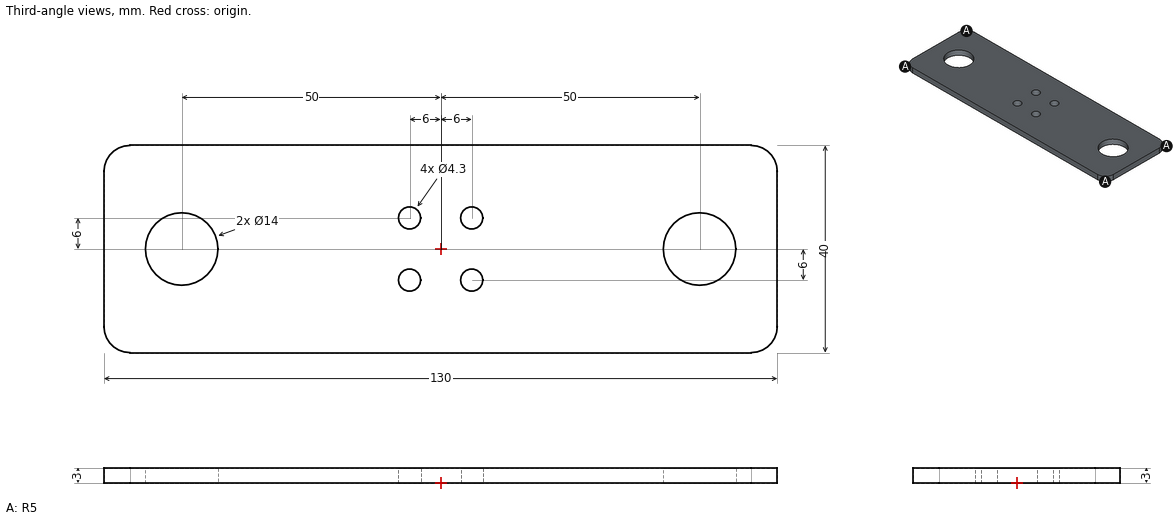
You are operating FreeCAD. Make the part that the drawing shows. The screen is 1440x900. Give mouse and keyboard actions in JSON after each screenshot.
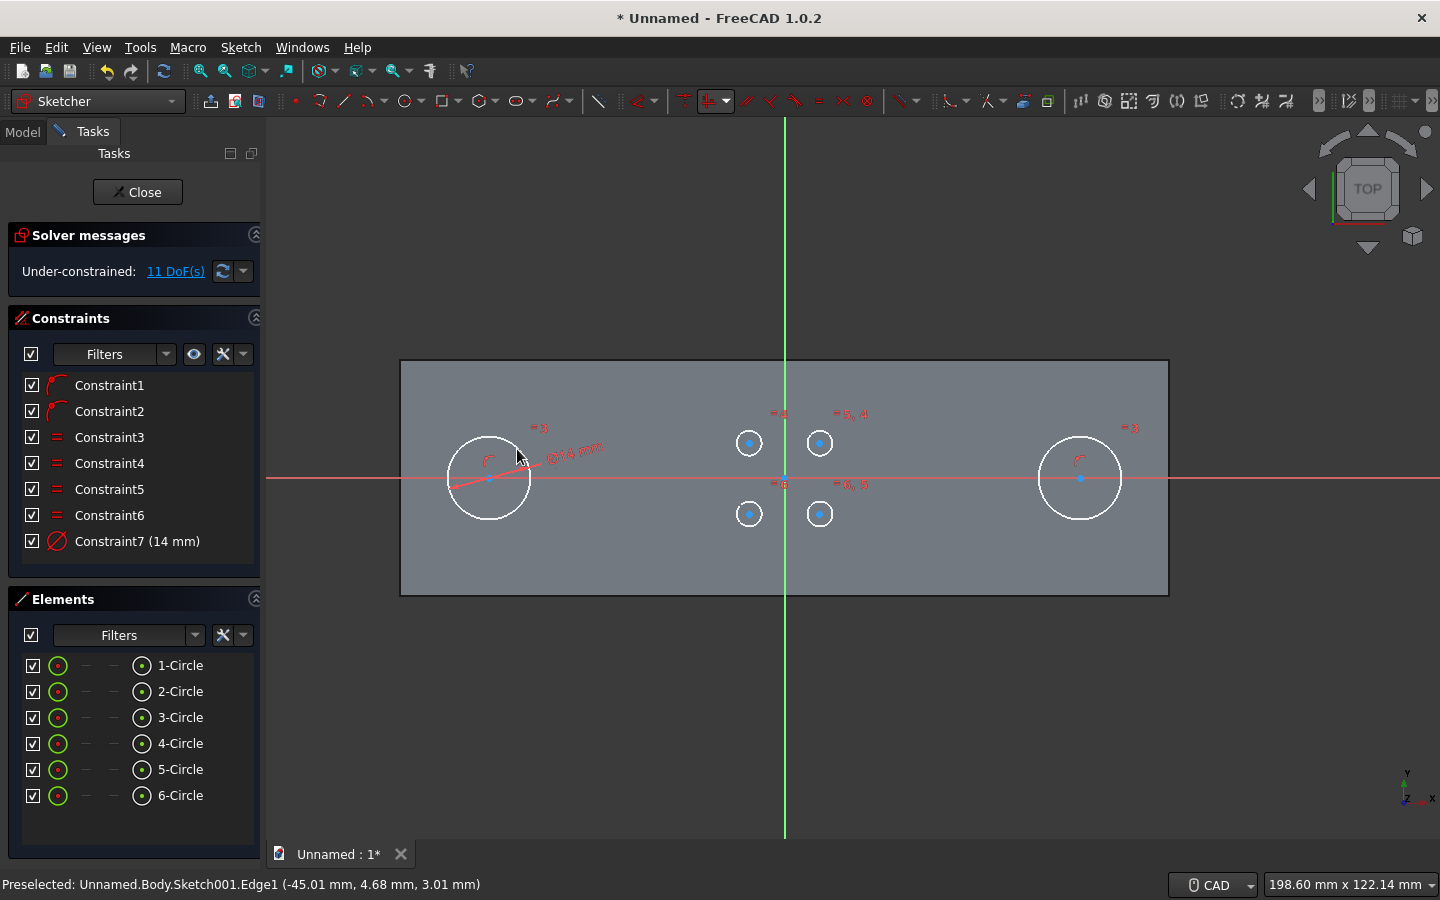
{"action": "scroll", "coordinate": [758, 434], "scroll_direction": "up", "scroll_amount": 3}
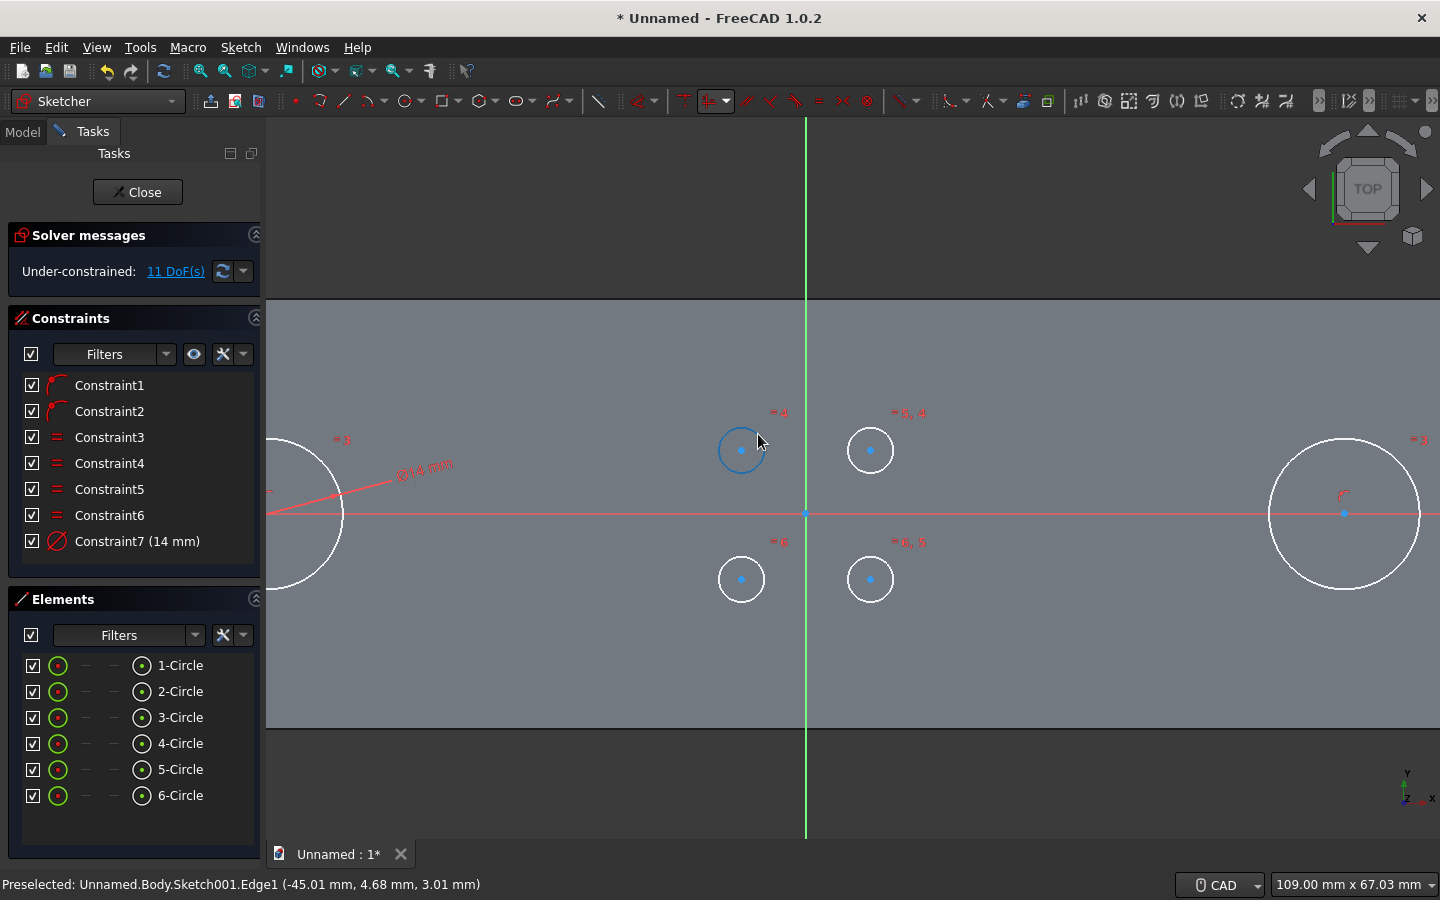
{"action": "left_click", "coordinate": [758, 434]}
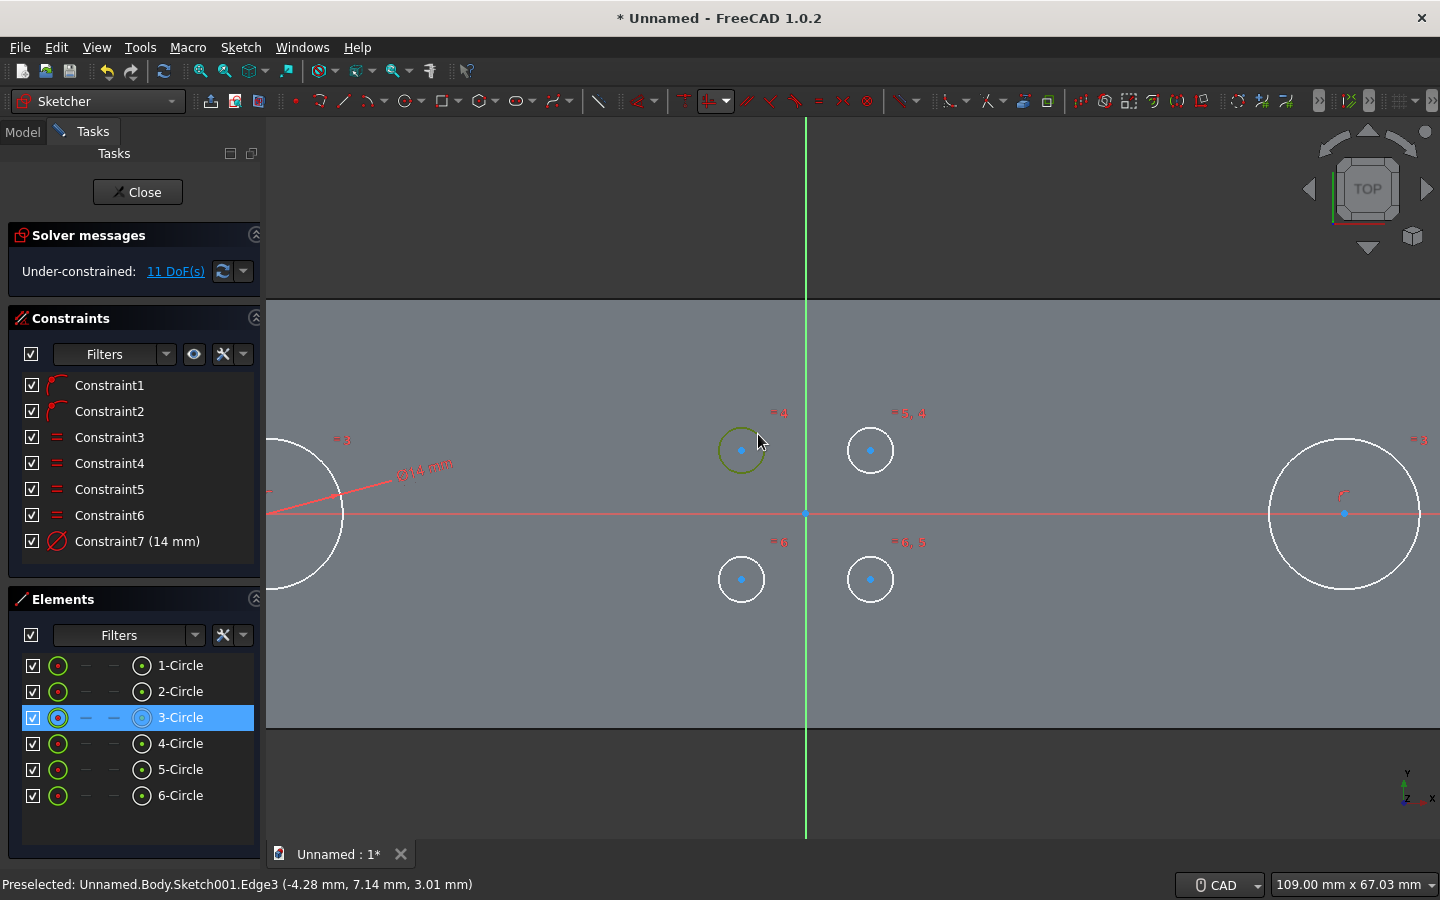
{"action": "key", "text": "k o"}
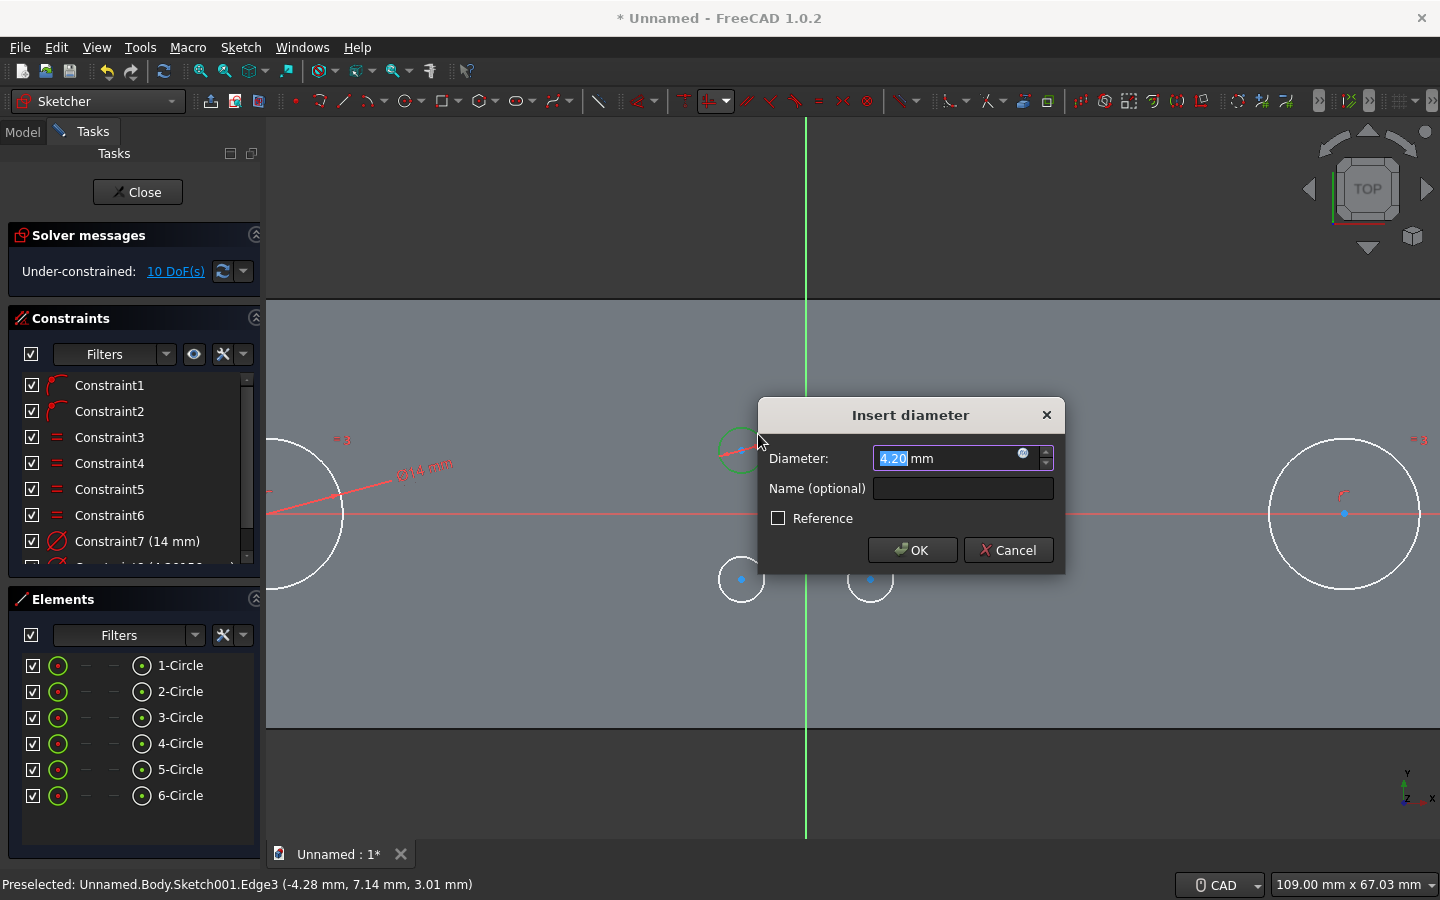
{"action": "type", "text": "4.3"}
{"action": "key", "text": "Return"}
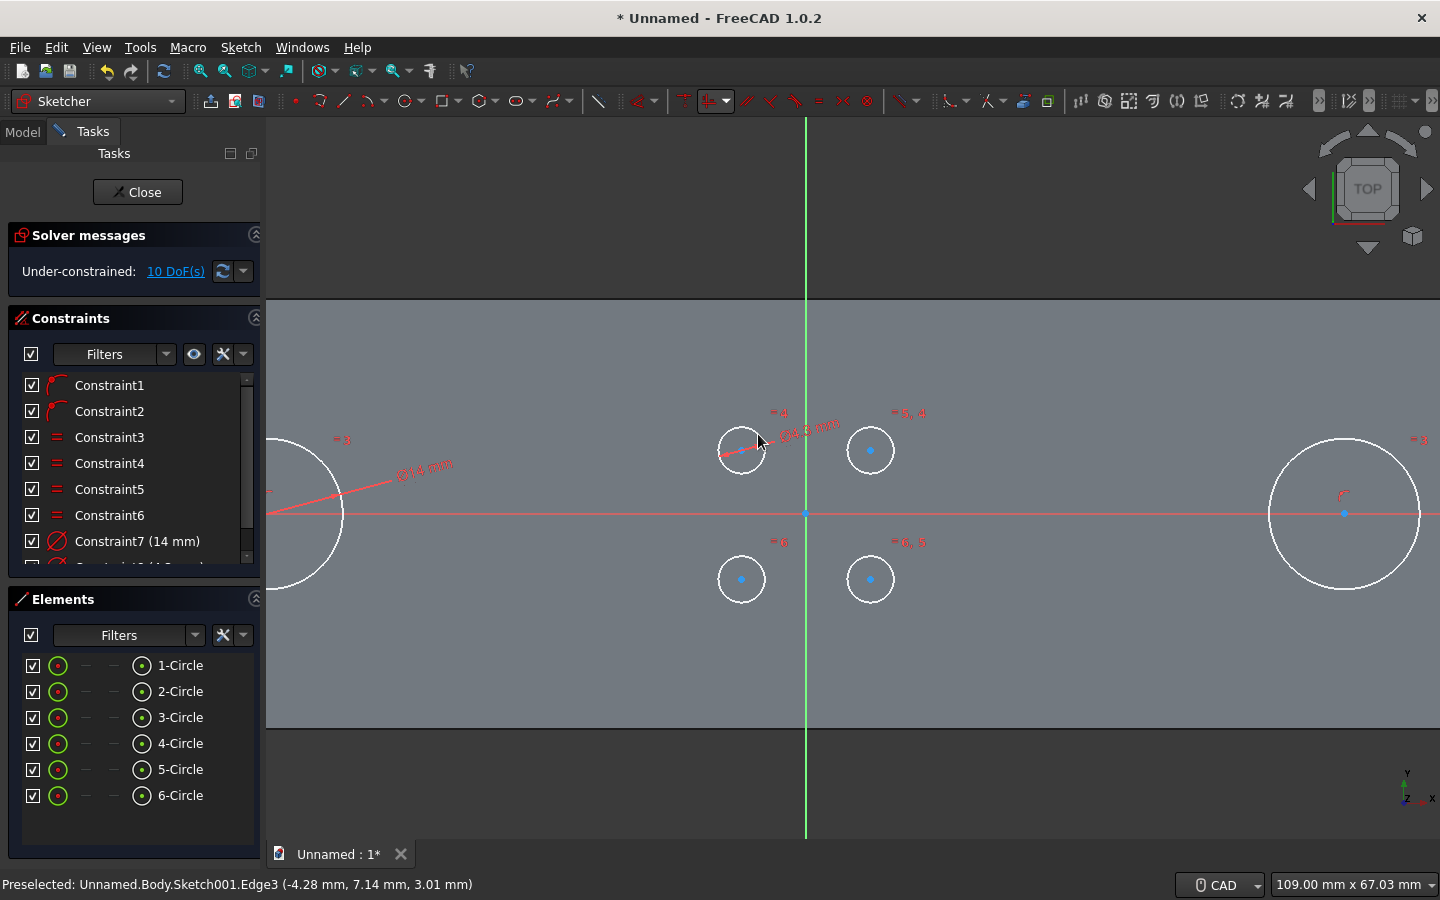
{"action": "left_click", "coordinate": [742, 450]}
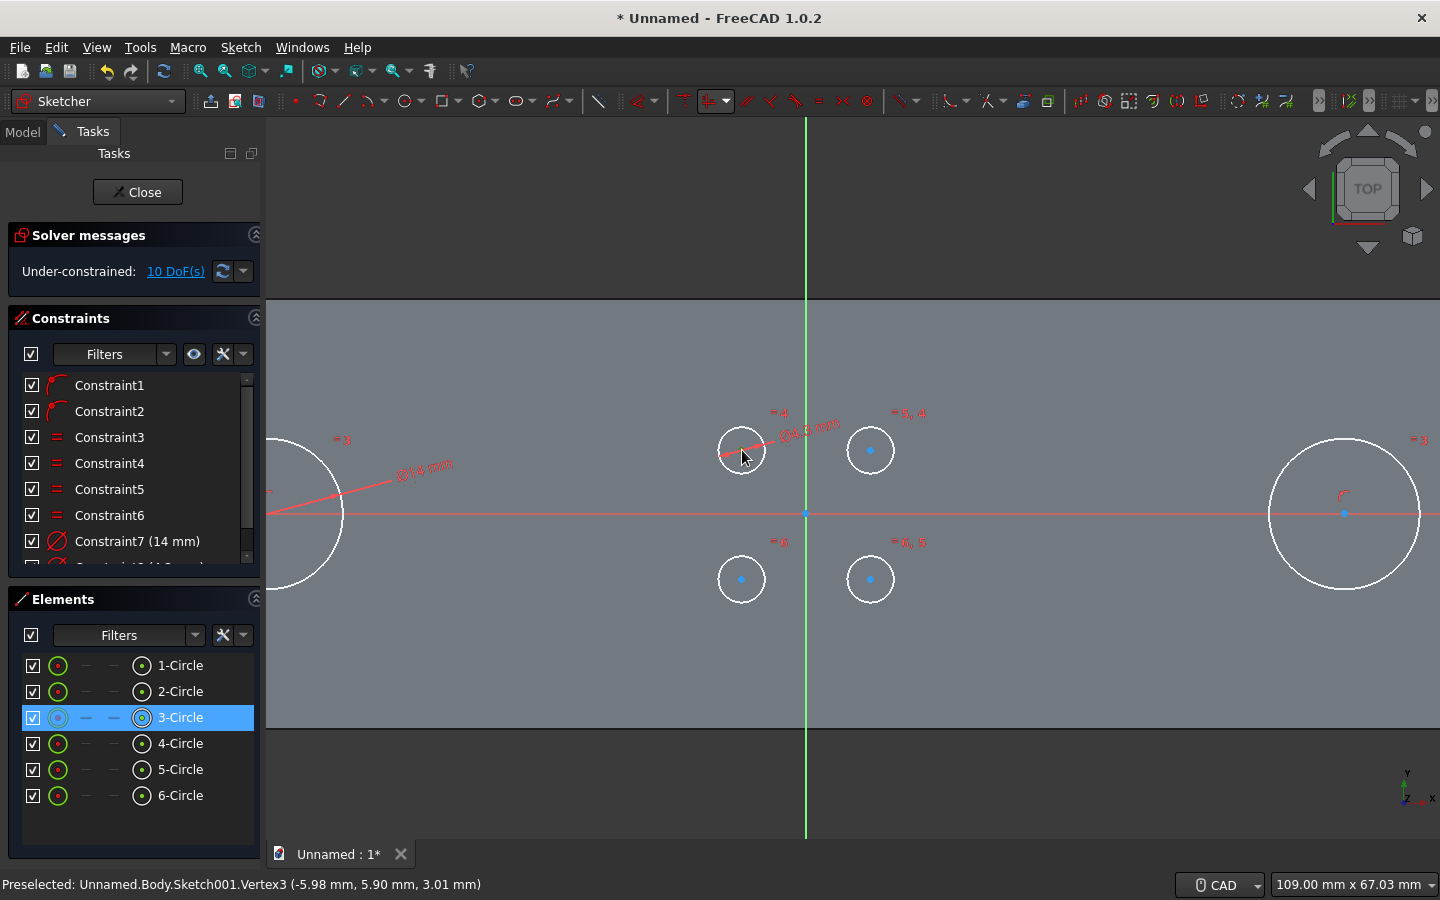
{"action": "key", "text": "l"}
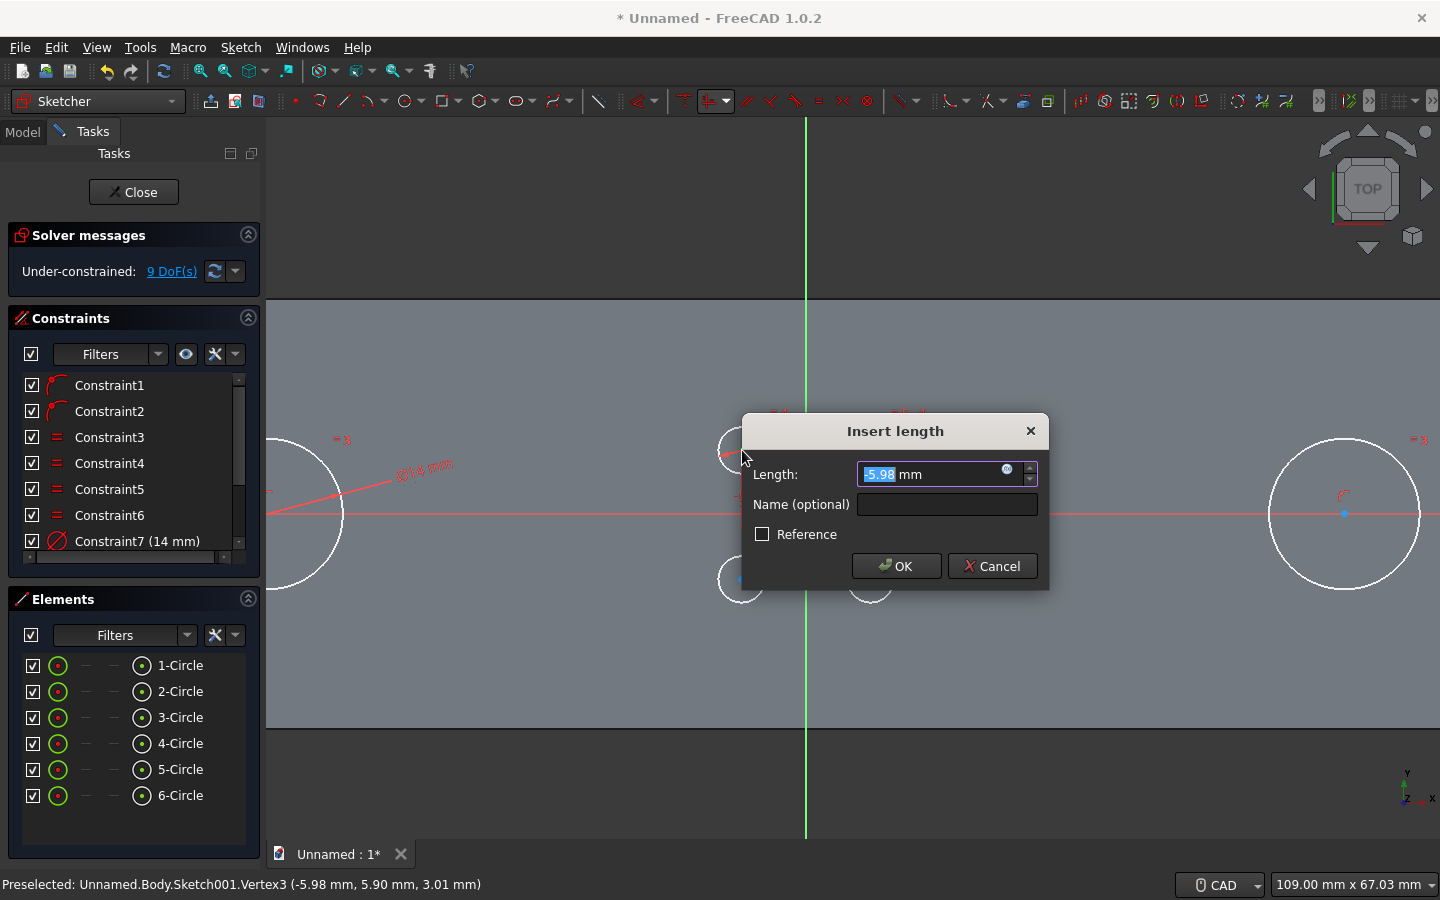
{"action": "type", "text": "-6"}
{"action": "key", "text": "Return"}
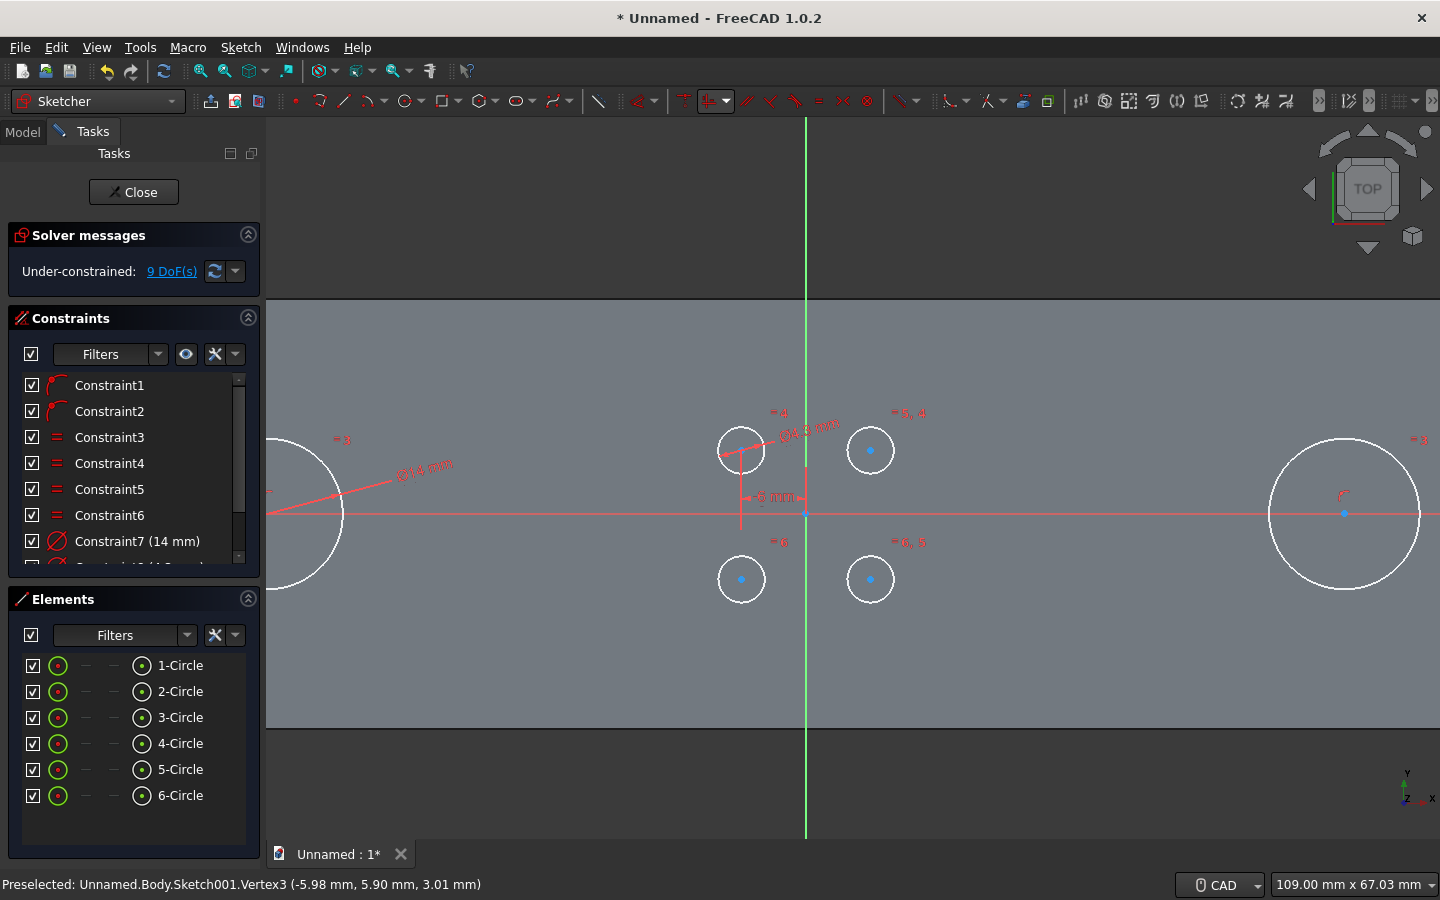
{"action": "left_click", "coordinate": [741, 450]}